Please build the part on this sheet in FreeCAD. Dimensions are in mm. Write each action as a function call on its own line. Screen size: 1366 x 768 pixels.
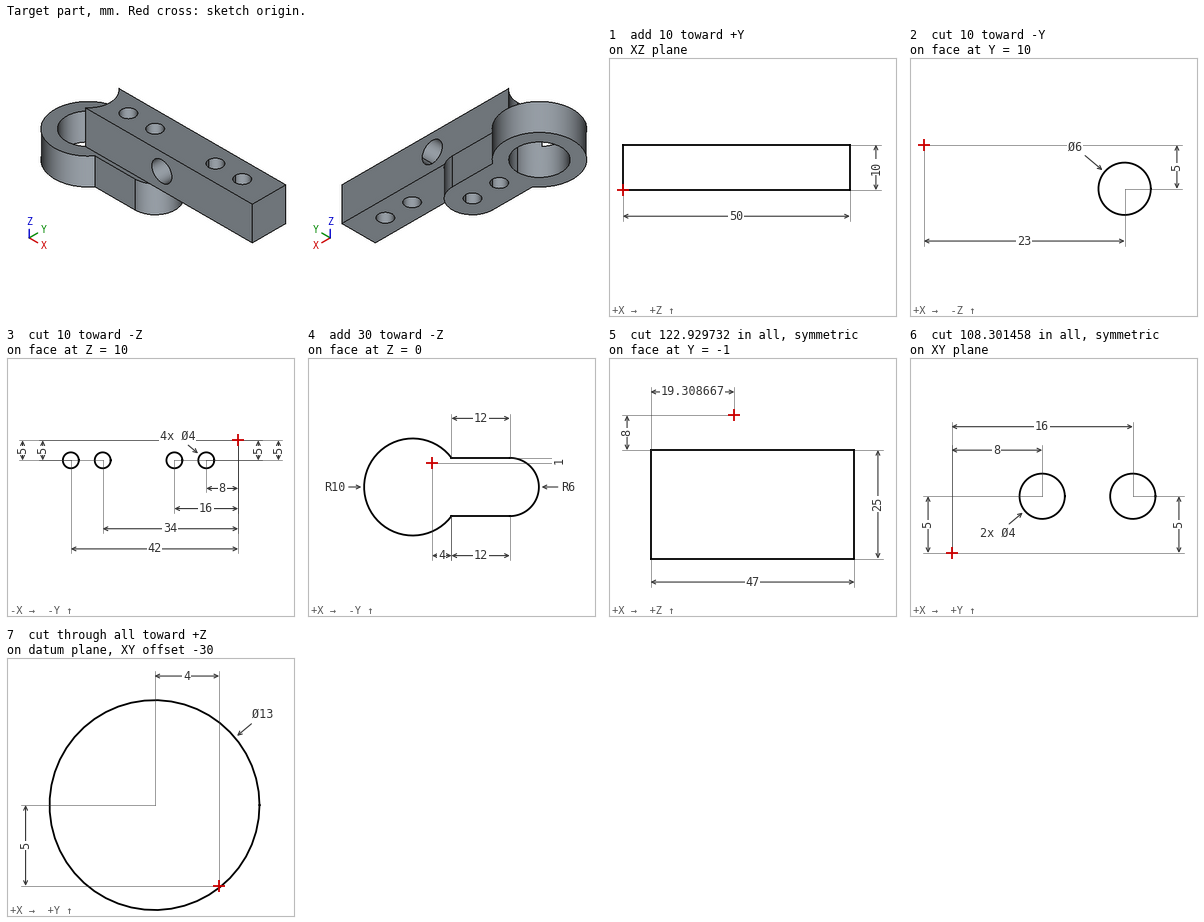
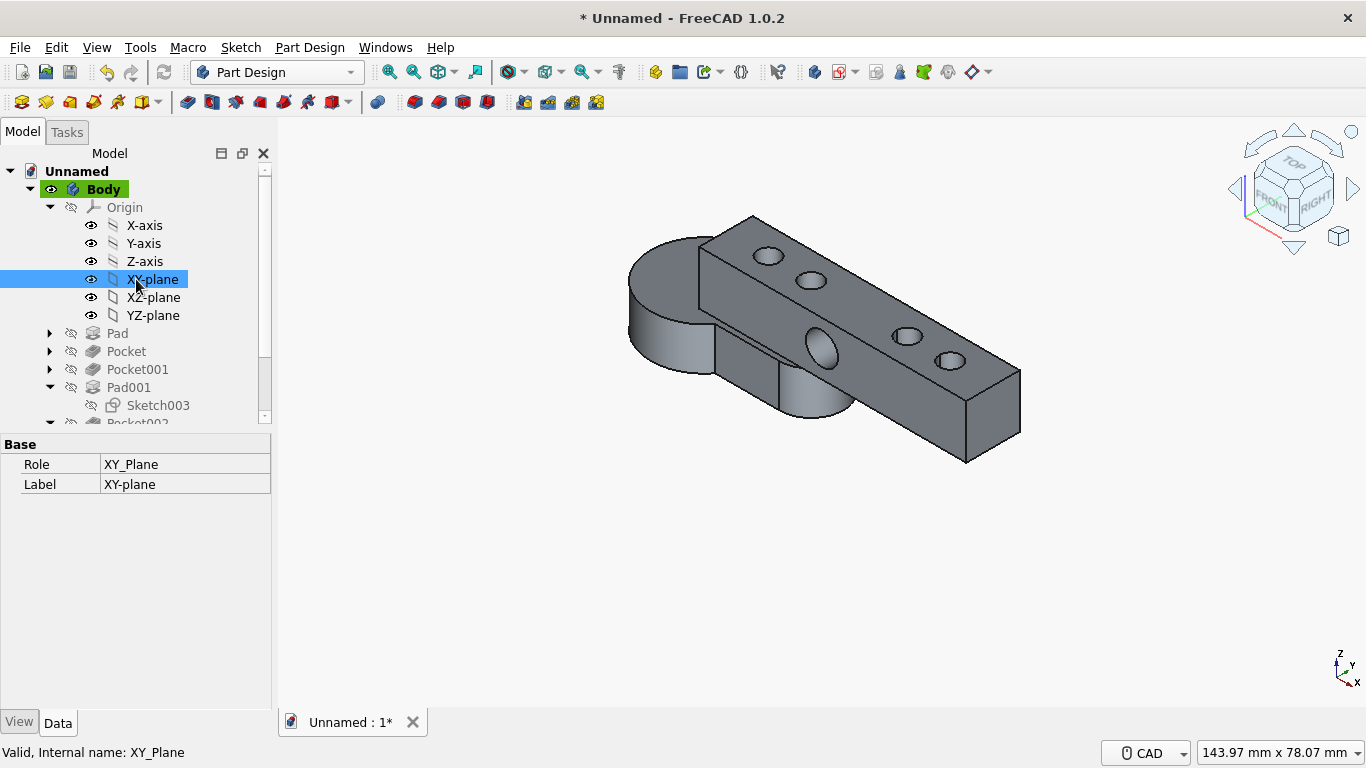
click(972, 72)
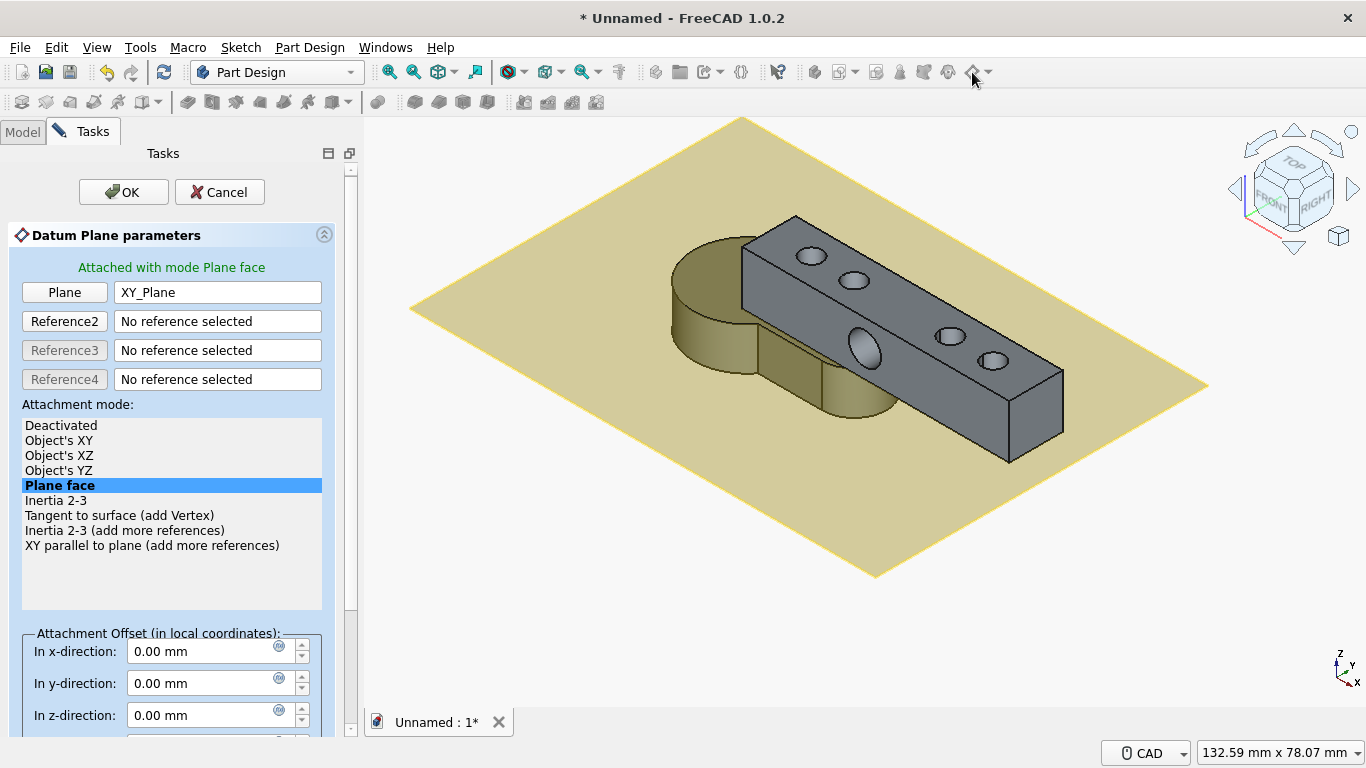
triple_click(210, 715)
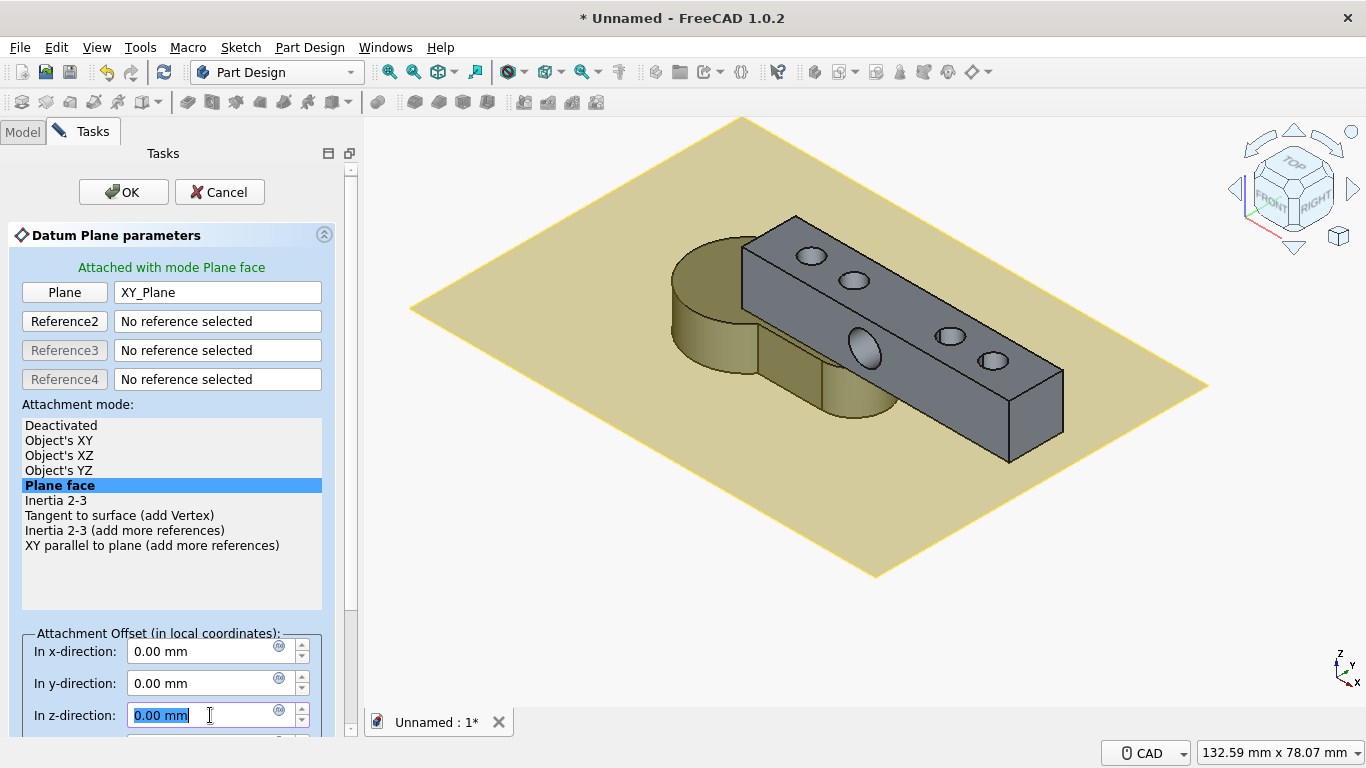
text(-30)
key(Tab)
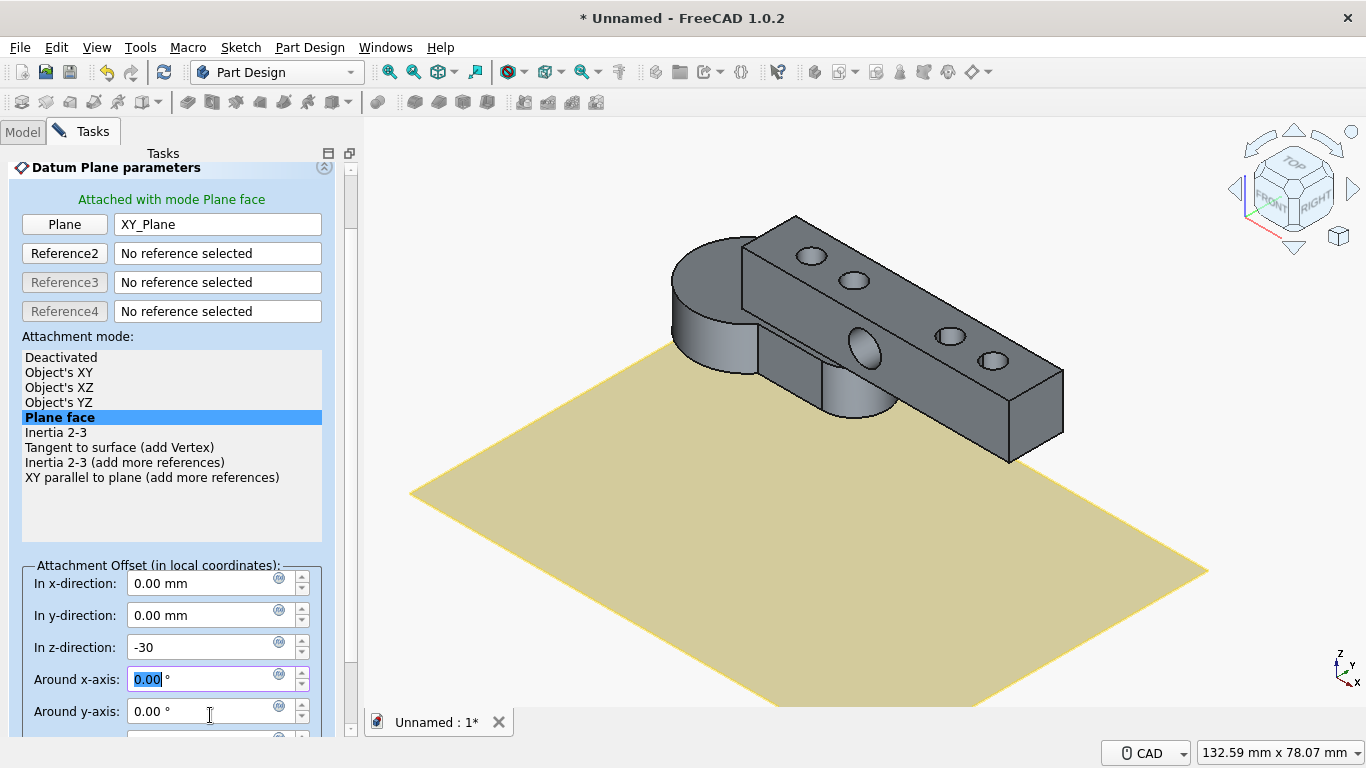
scroll(351, 450, up, 2)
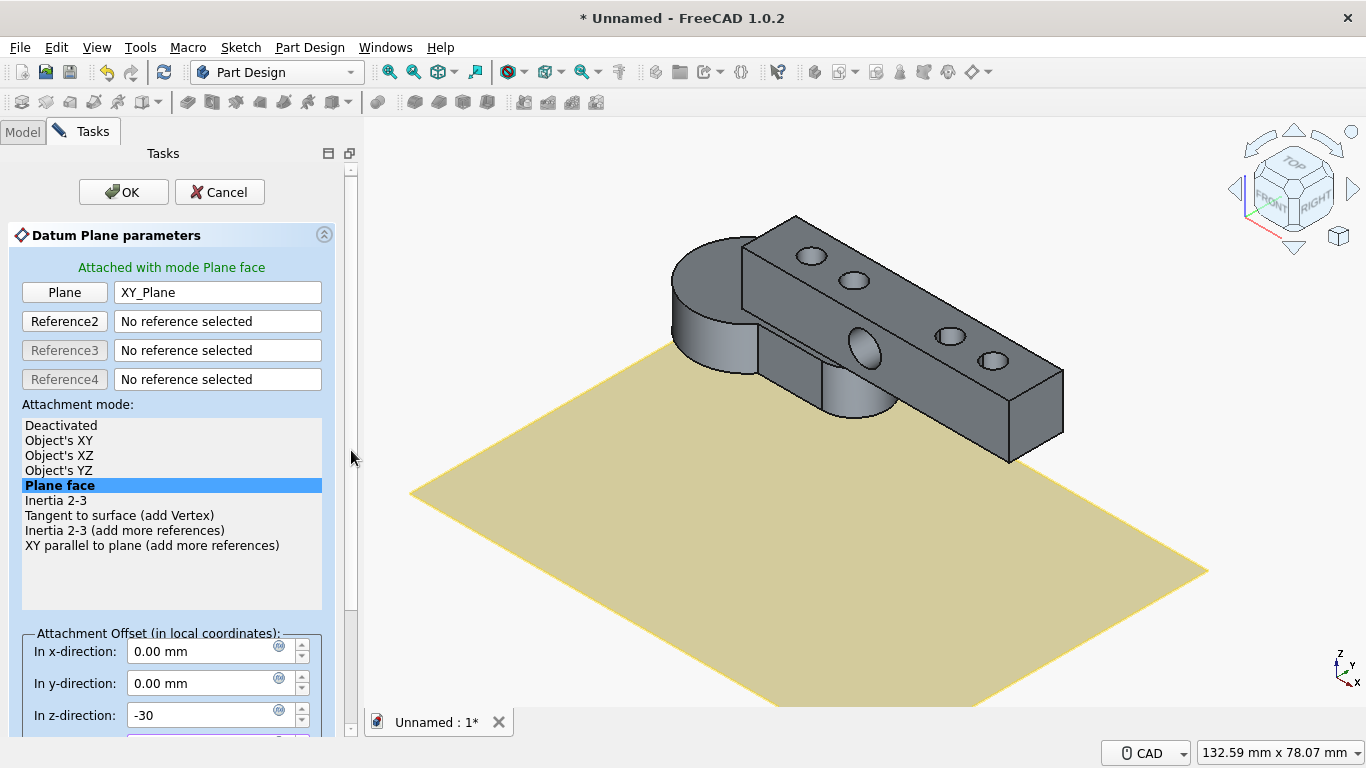
click(124, 192)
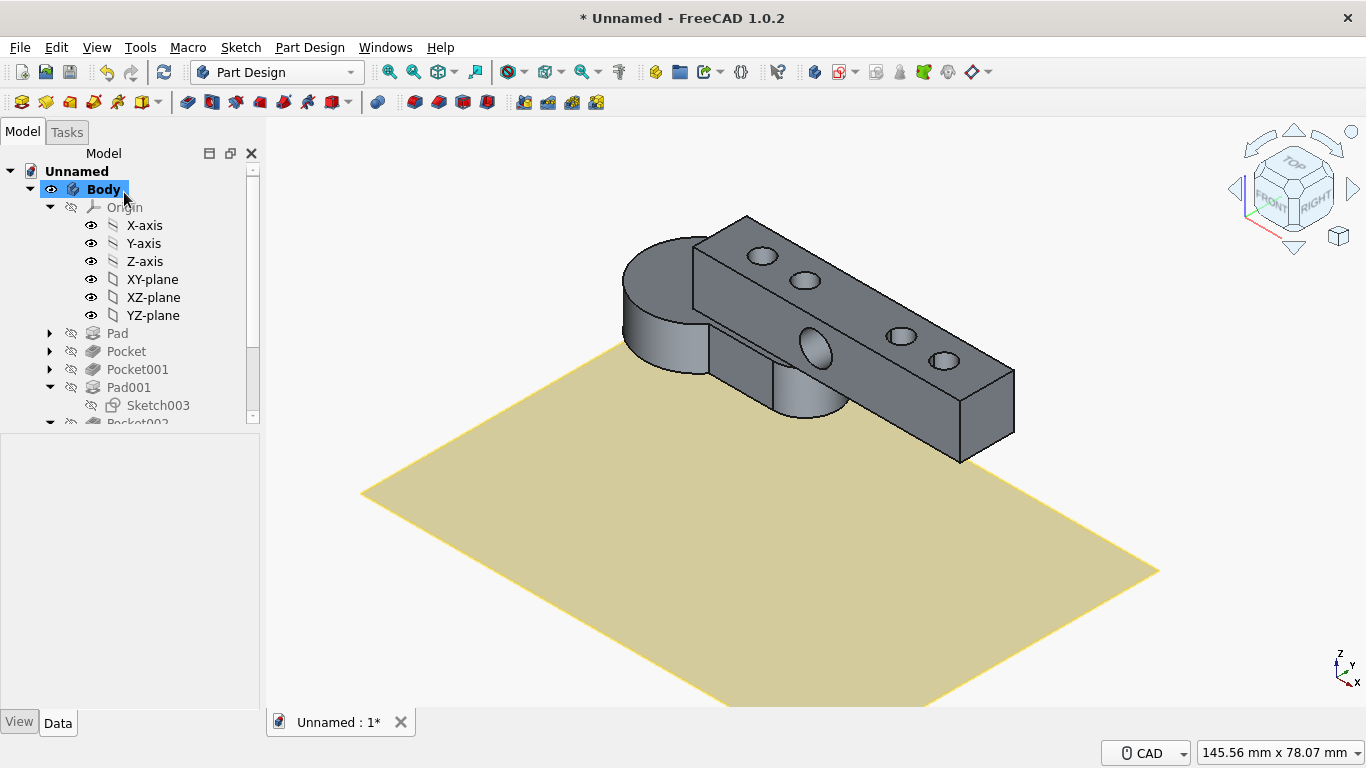
scroll(100, 293, down, 3)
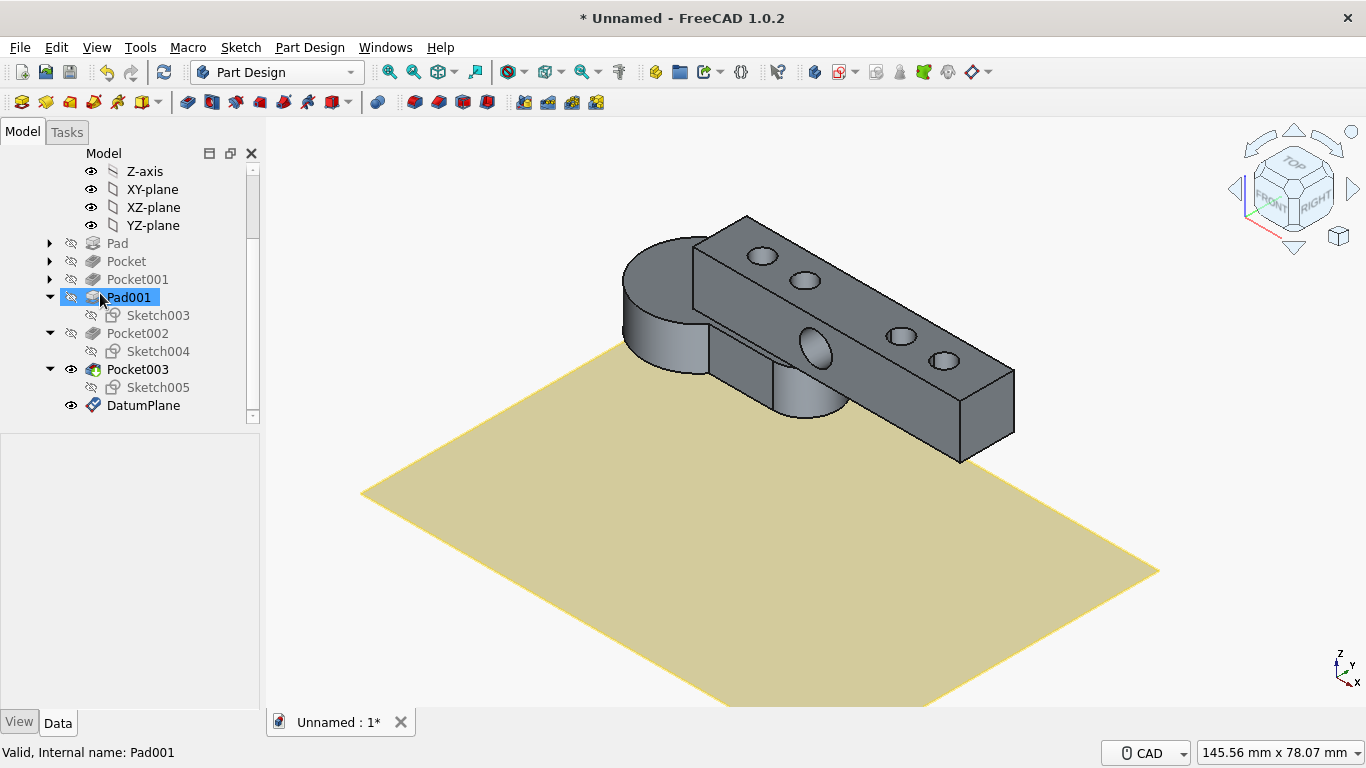
click(116, 405)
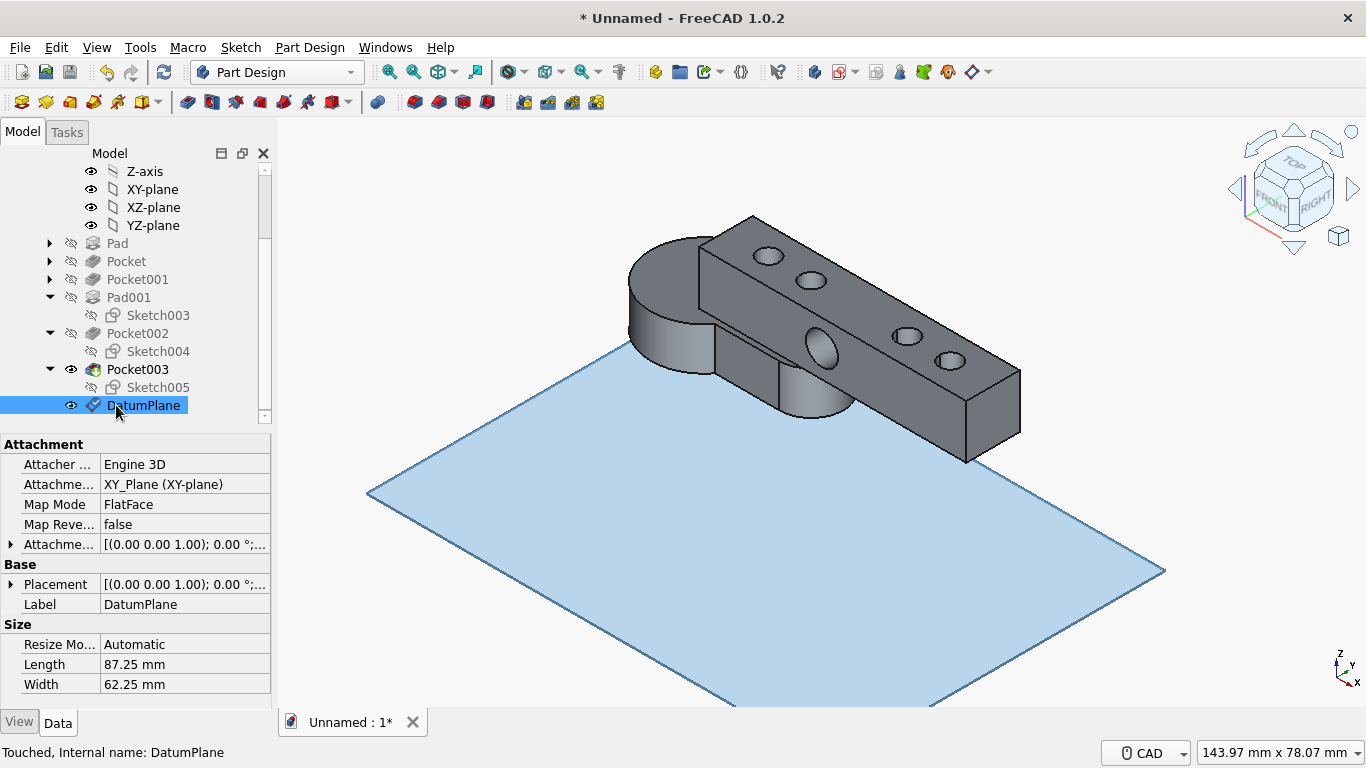
click(840, 72)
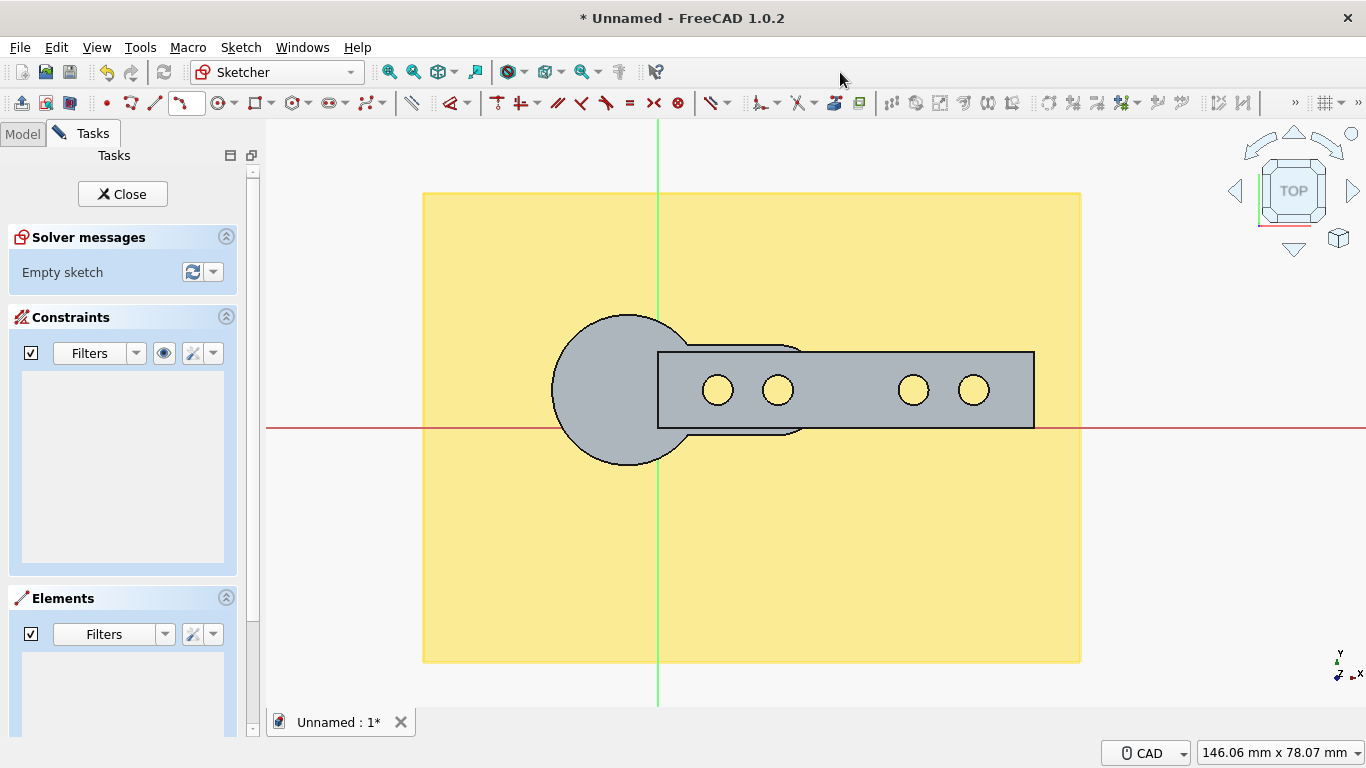
click(70, 104)